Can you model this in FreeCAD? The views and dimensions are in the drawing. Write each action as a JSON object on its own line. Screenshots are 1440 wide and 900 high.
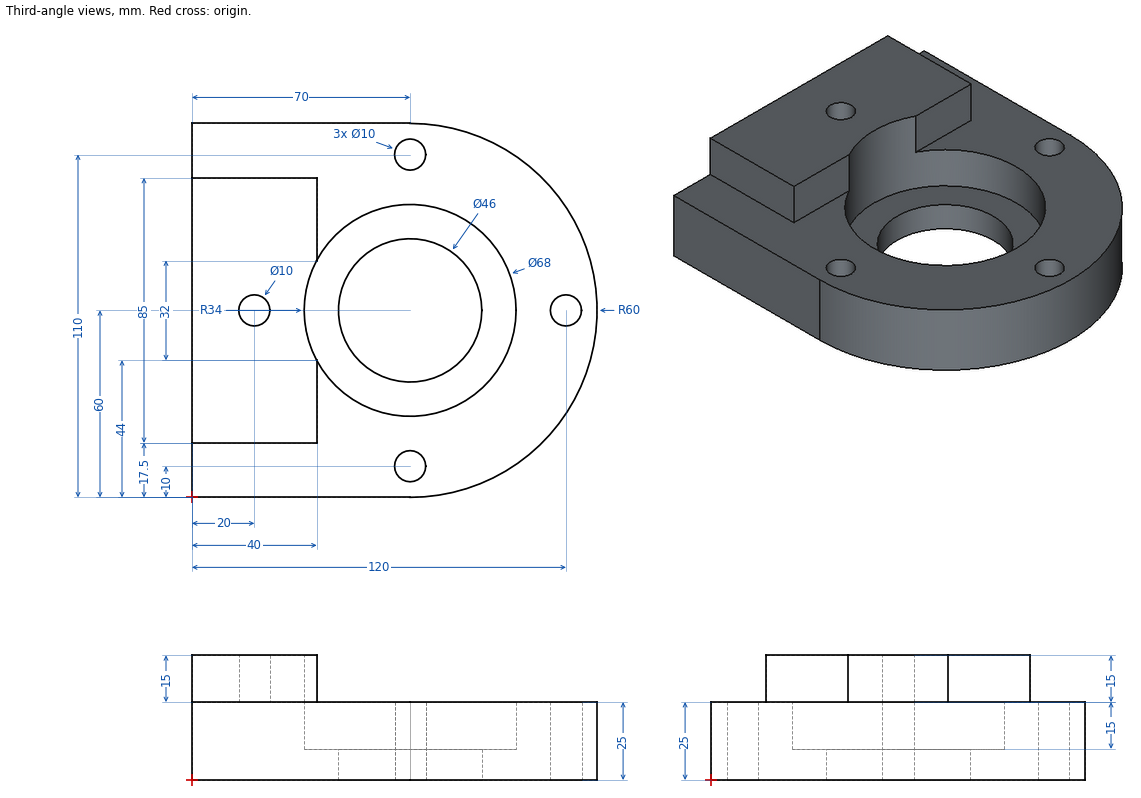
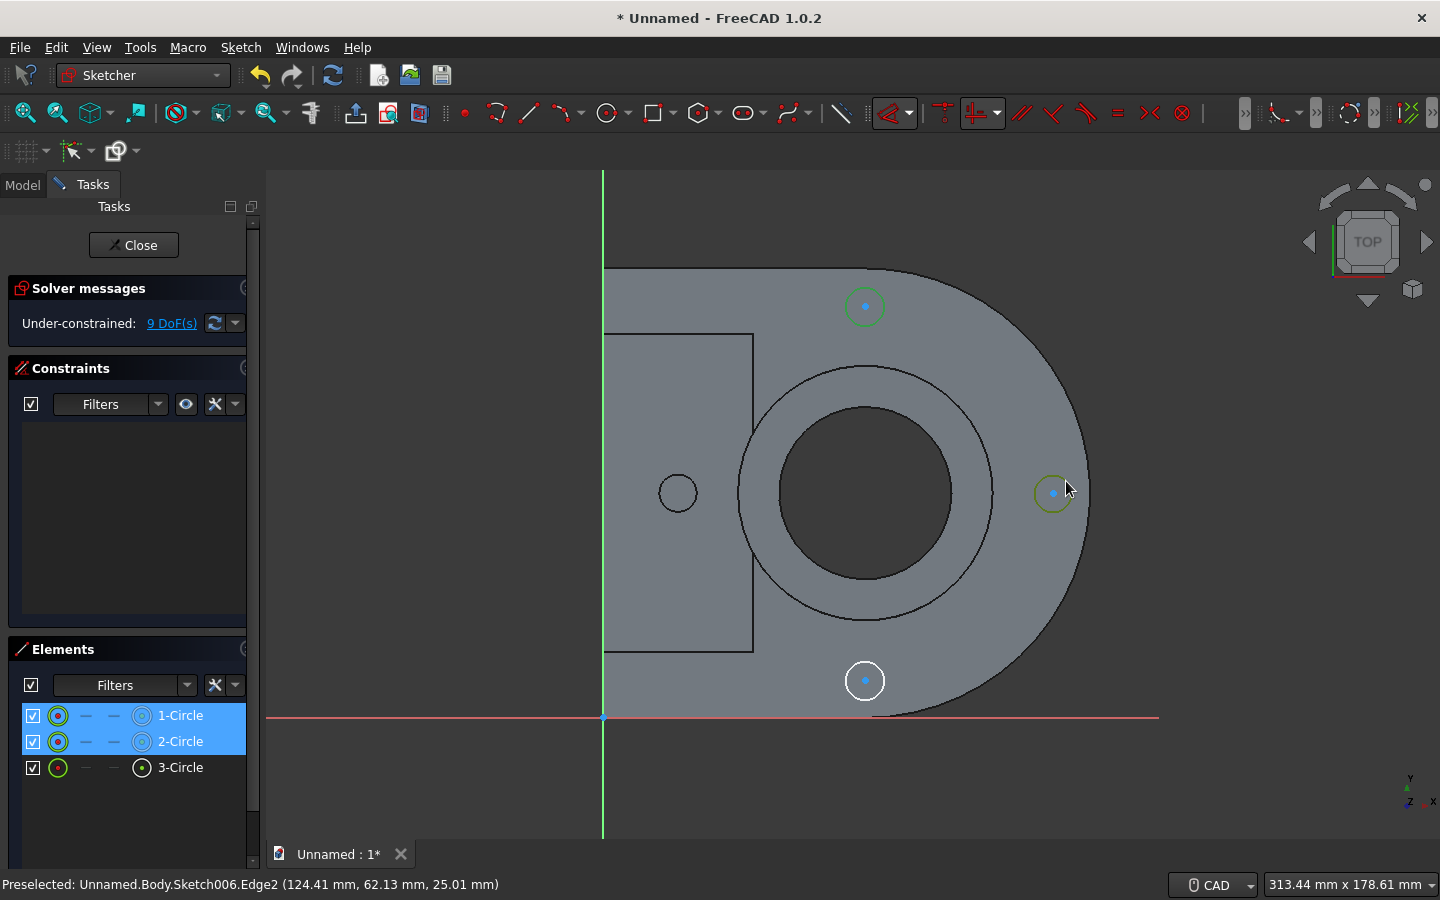
{"action": "left_click", "coordinate": [878, 667]}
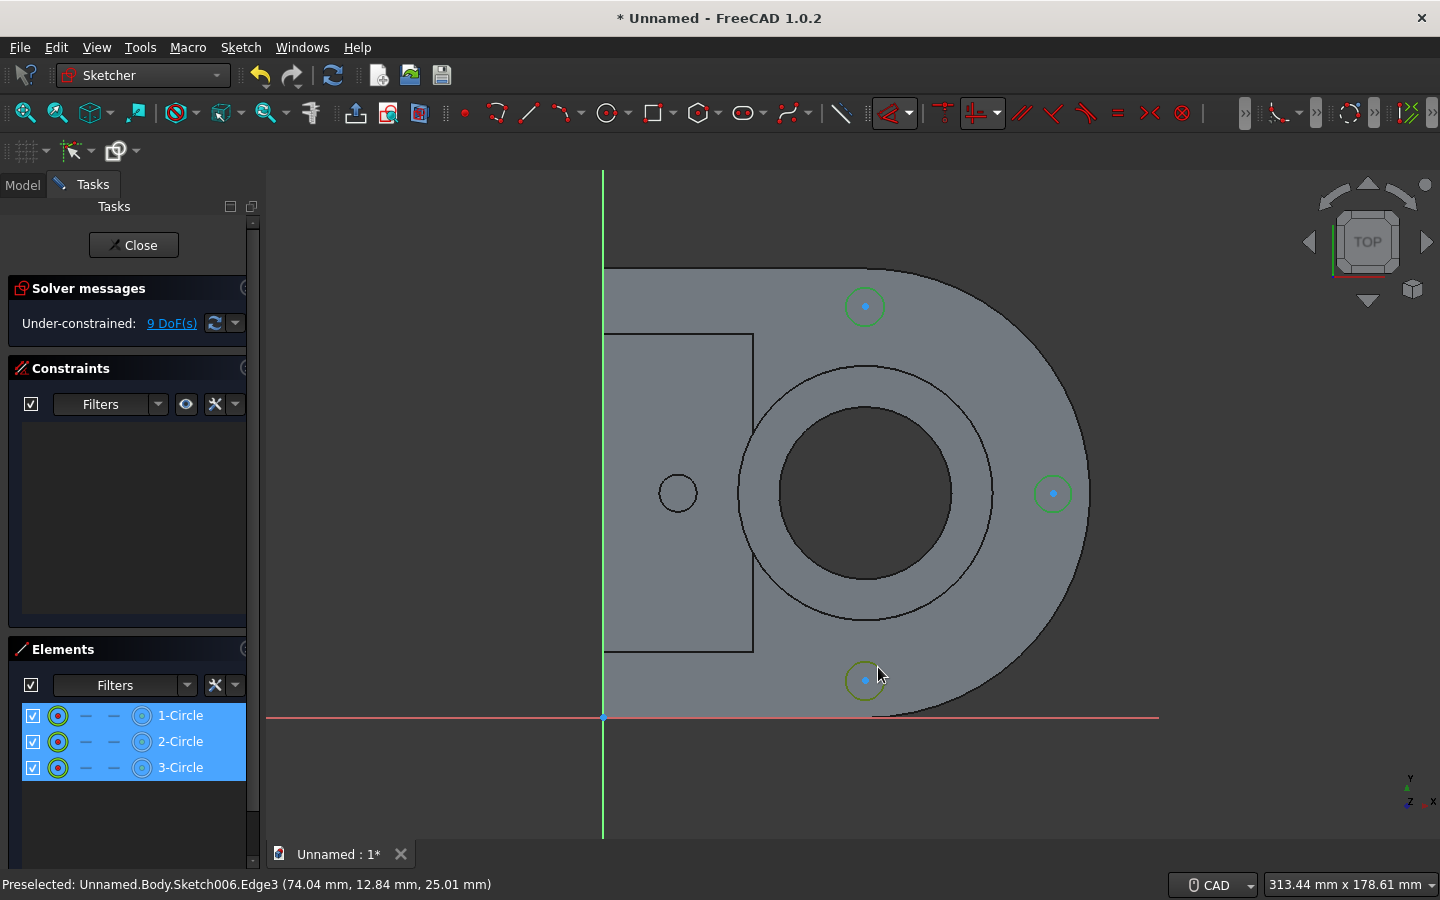
{"action": "left_click", "coordinate": [1118, 114]}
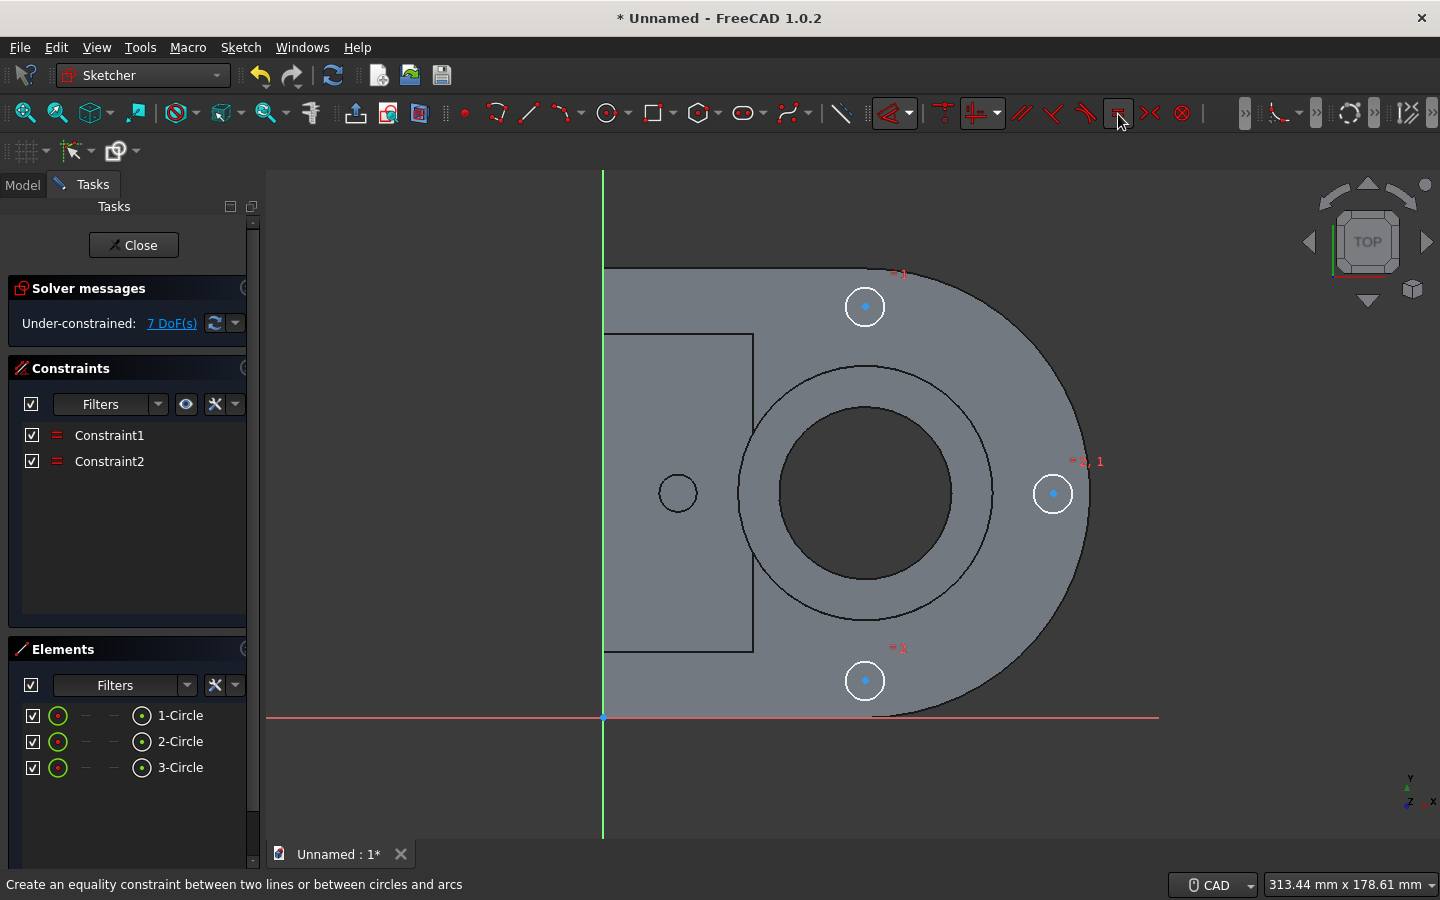
{"action": "left_click", "coordinate": [878, 293]}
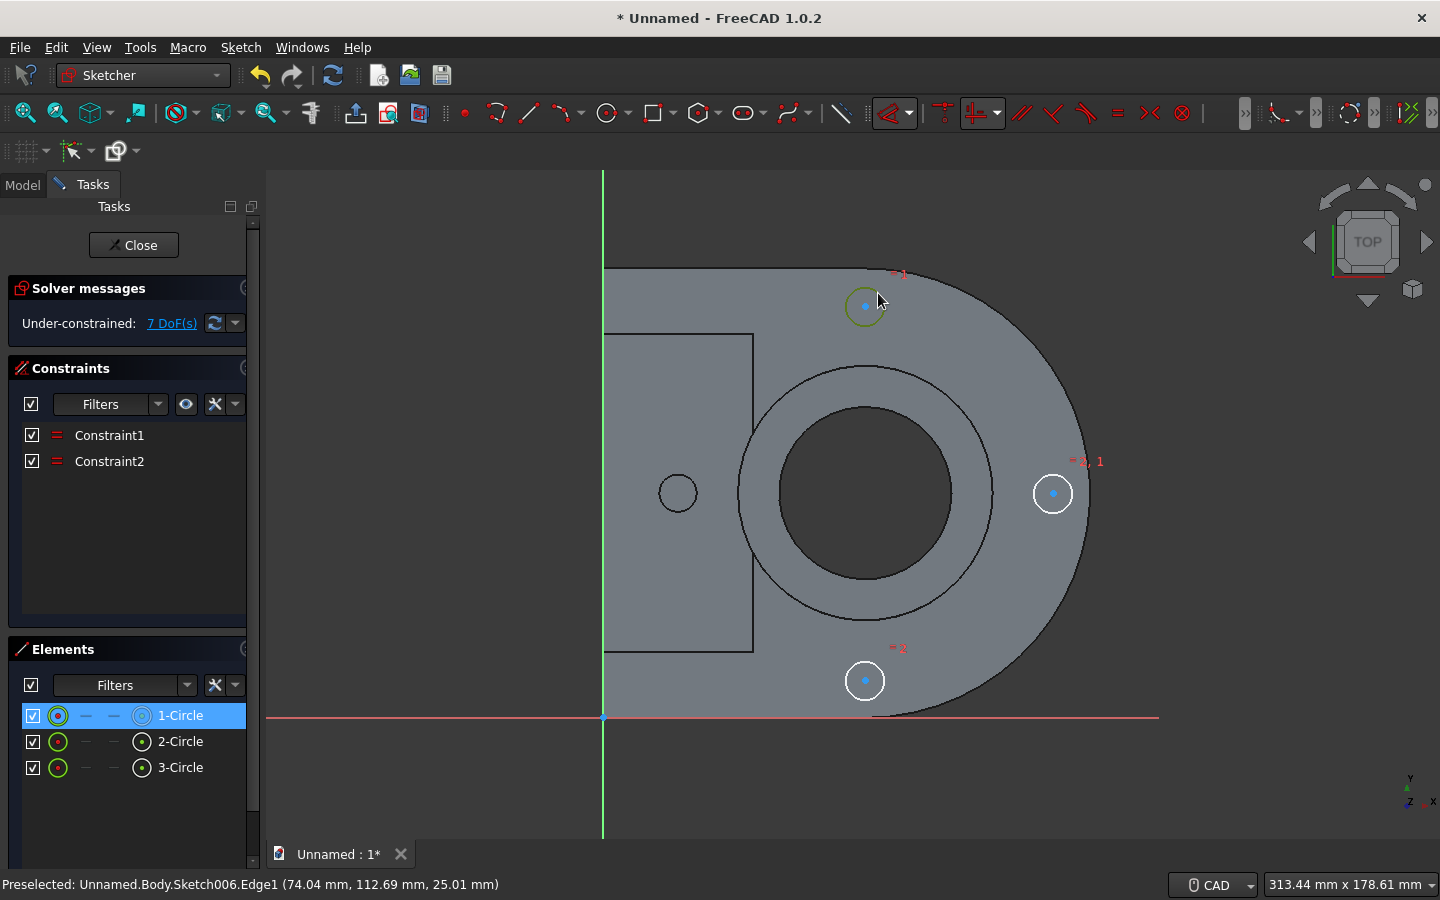
{"action": "left_click", "coordinate": [912, 114]}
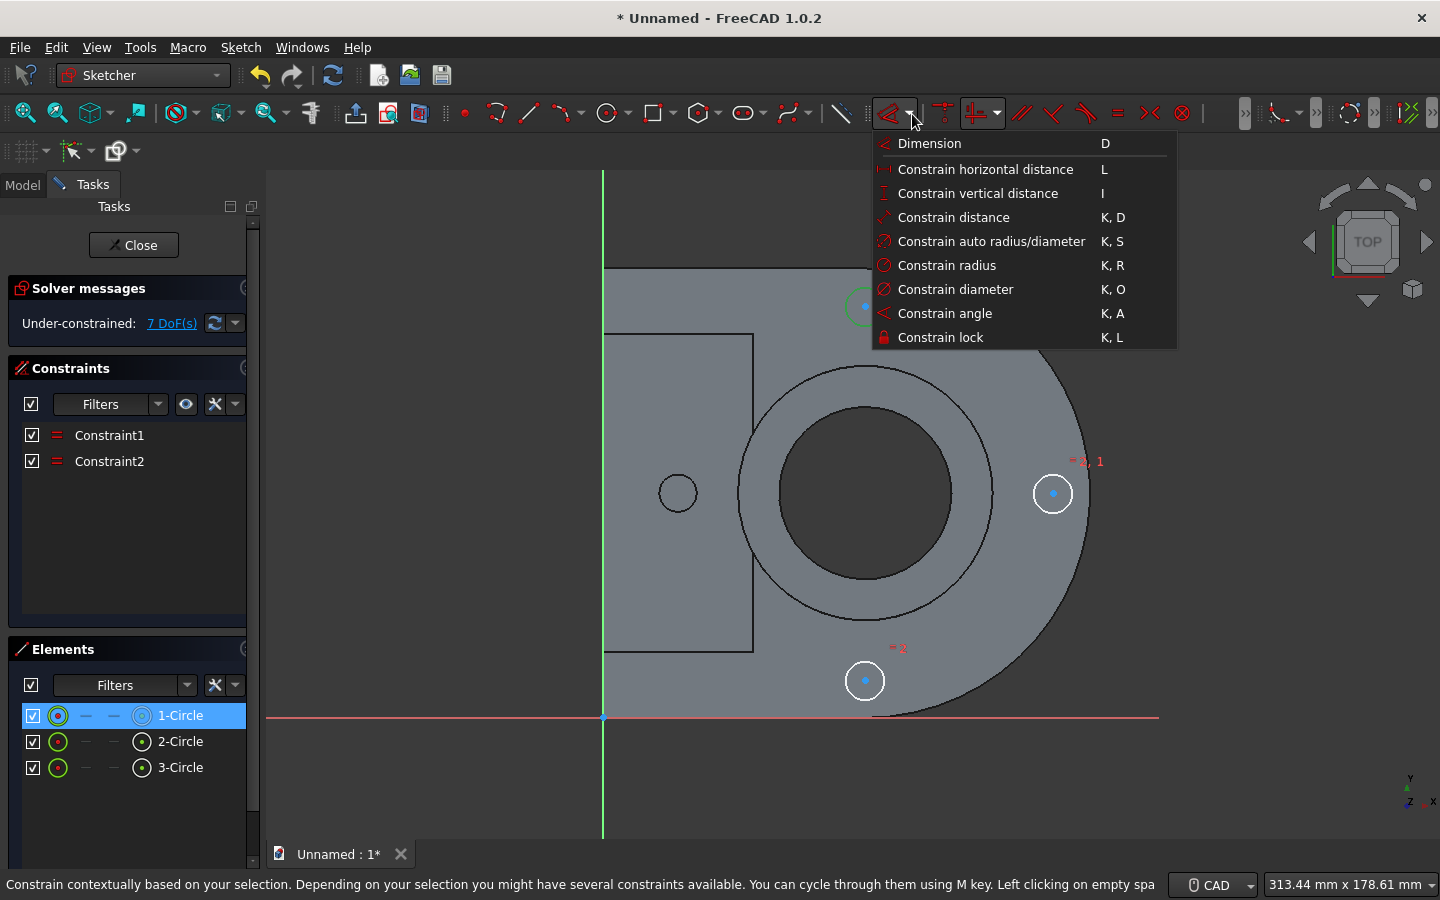
{"action": "left_click", "coordinate": [1025, 289]}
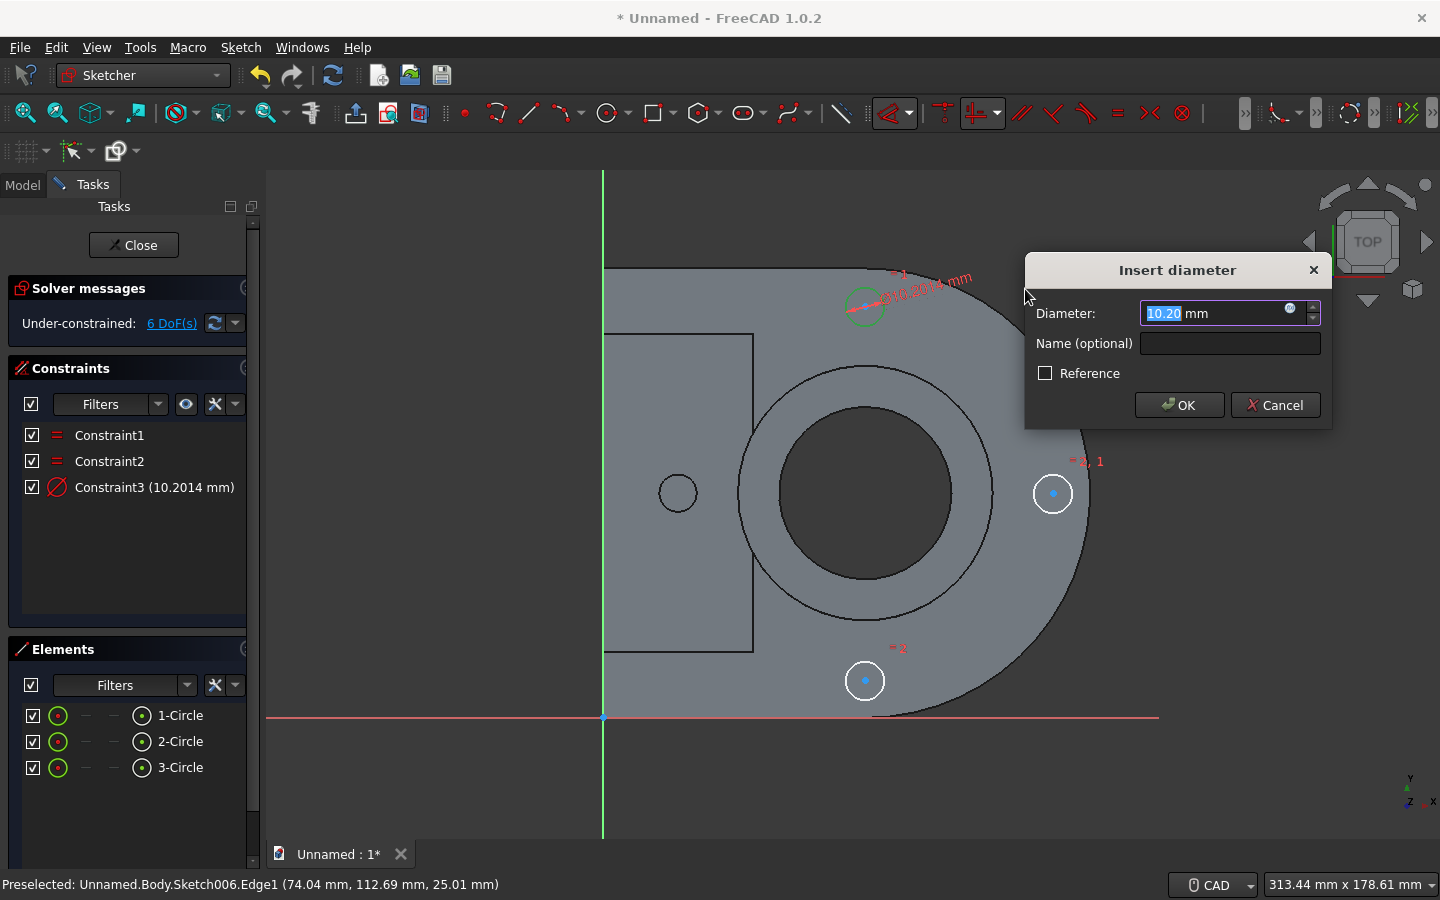
{"action": "type", "text": "10"}
{"action": "key", "text": "Return"}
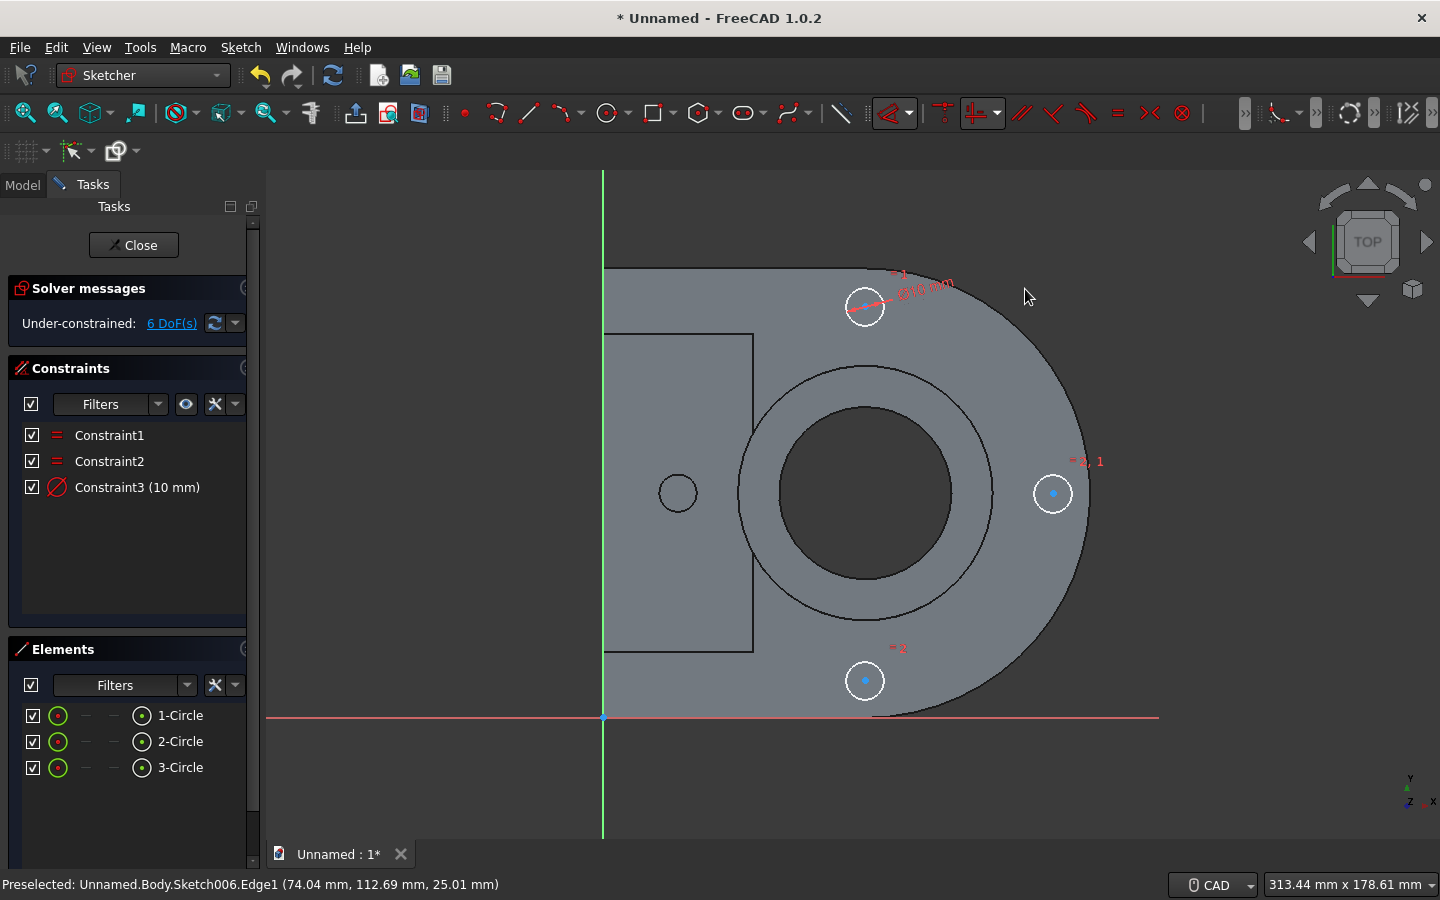
{"action": "left_click", "coordinate": [865, 307]}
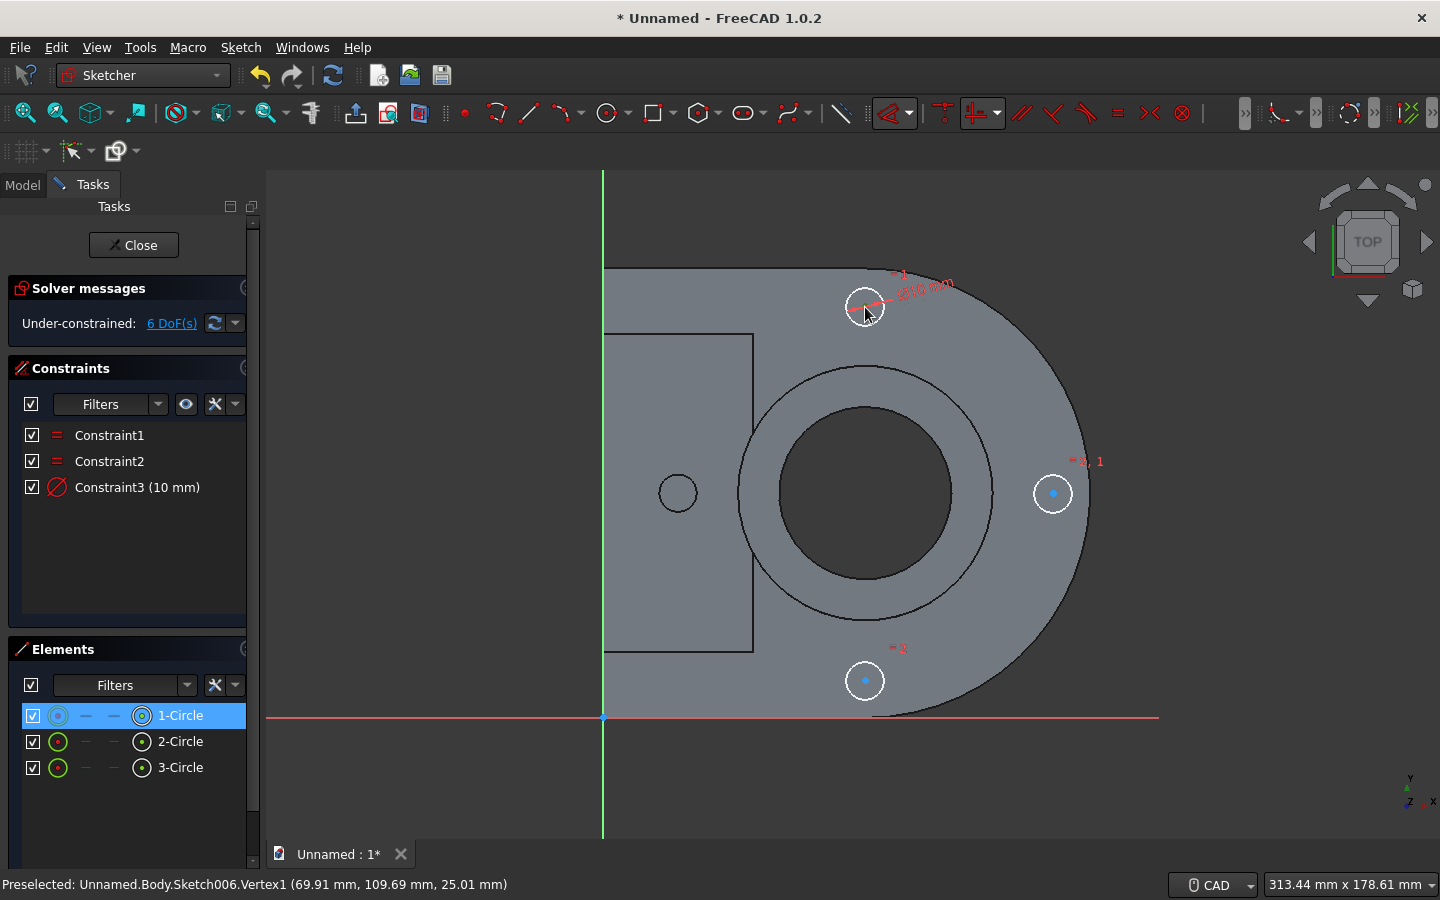
{"action": "key", "text": "l"}